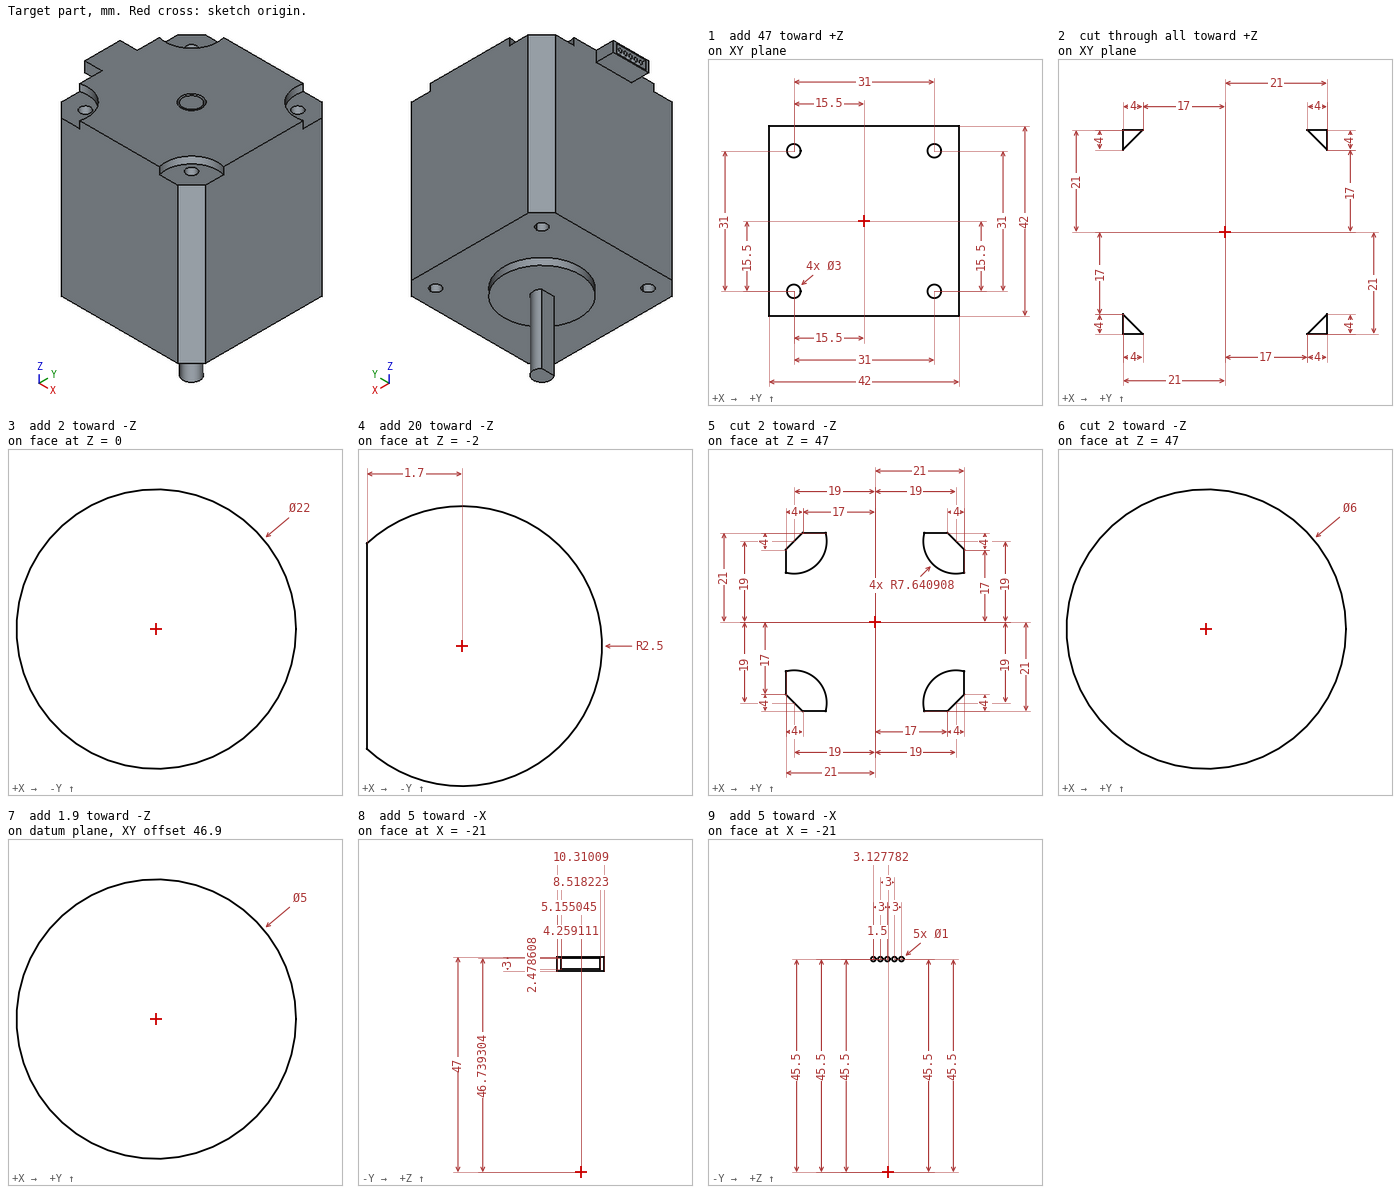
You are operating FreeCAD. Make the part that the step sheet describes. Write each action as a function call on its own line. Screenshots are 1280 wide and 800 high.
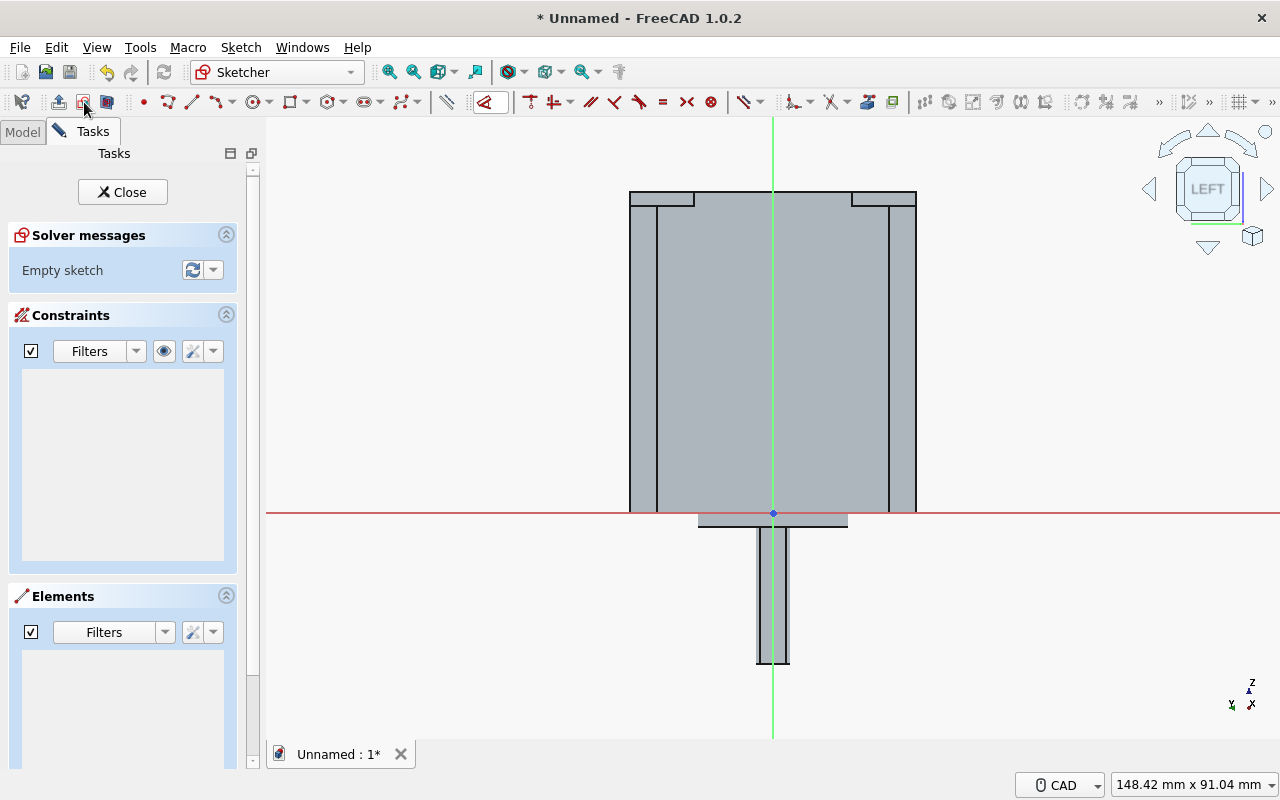
scroll(782, 174, up, 11)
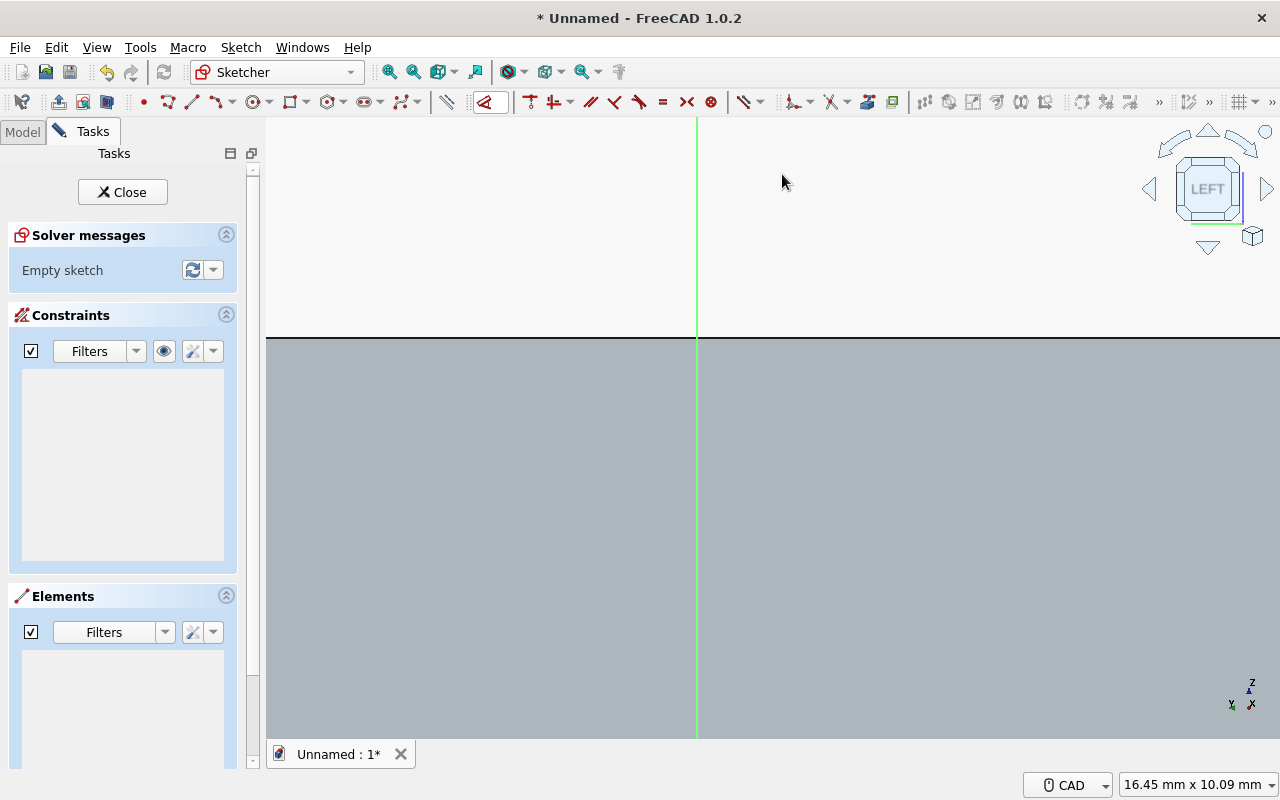
key(g)
key(r)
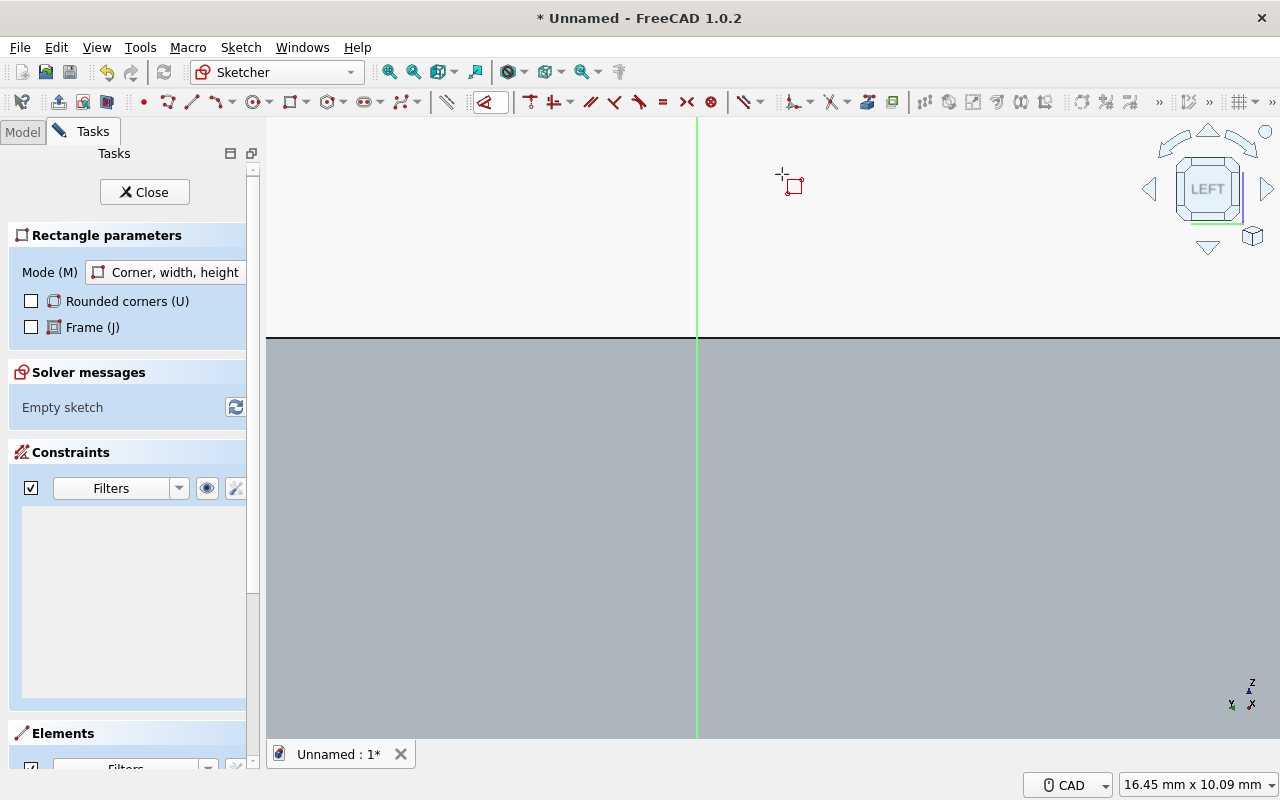
click(379, 338)
click(1015, 523)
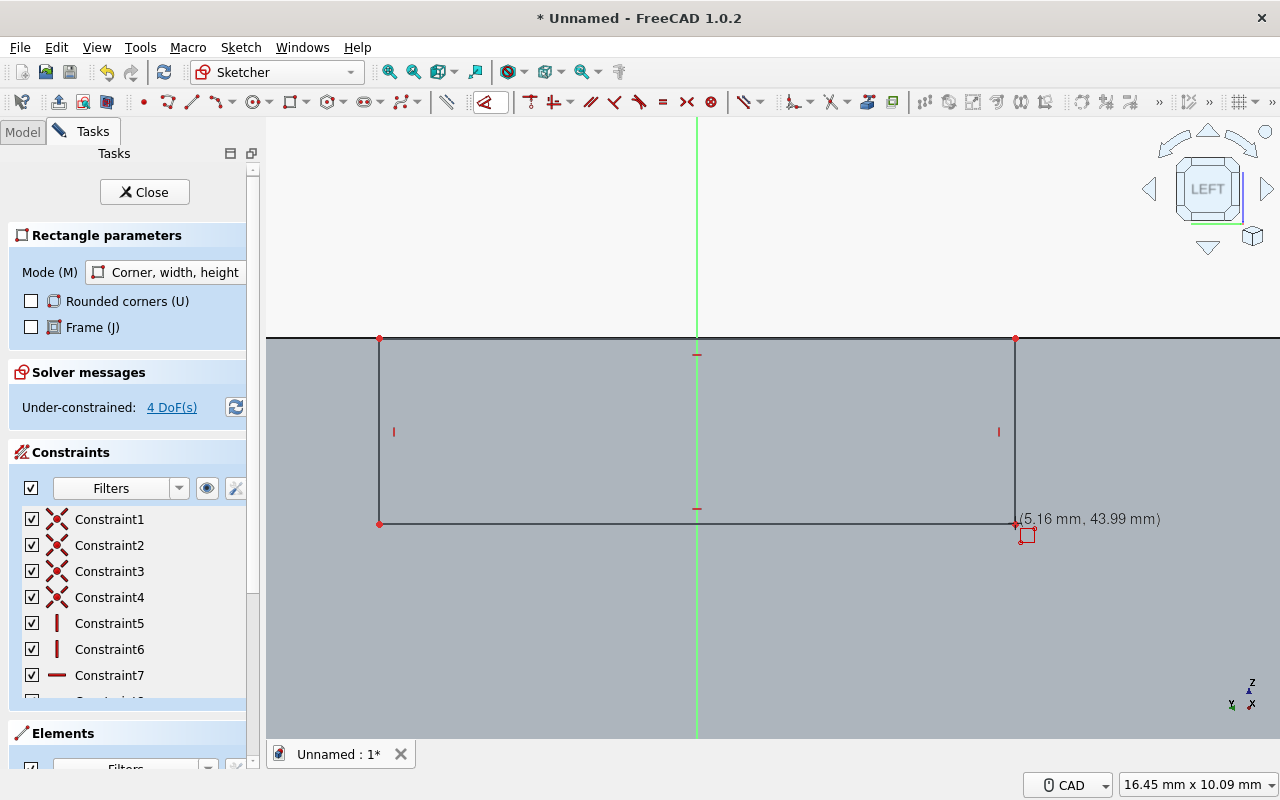
click(434, 355)
click(959, 507)
key(Escape)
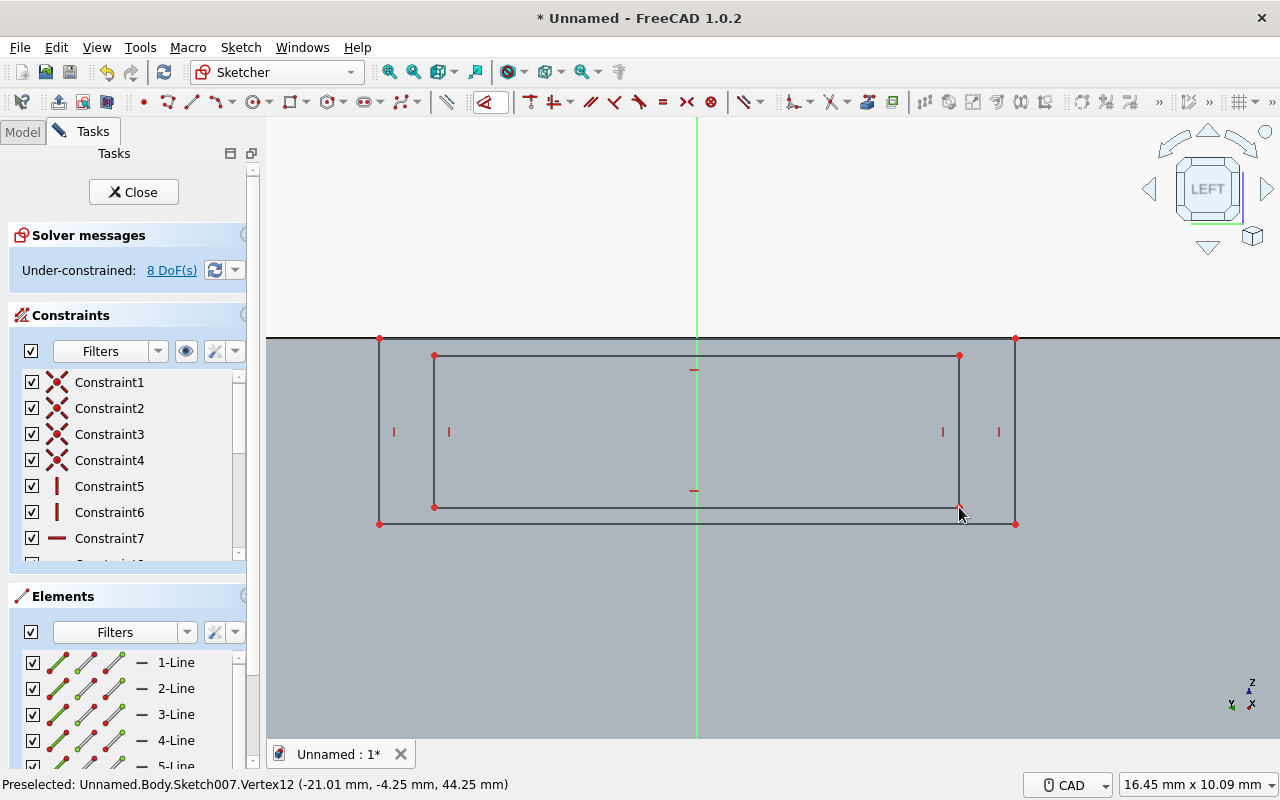
click(379, 394)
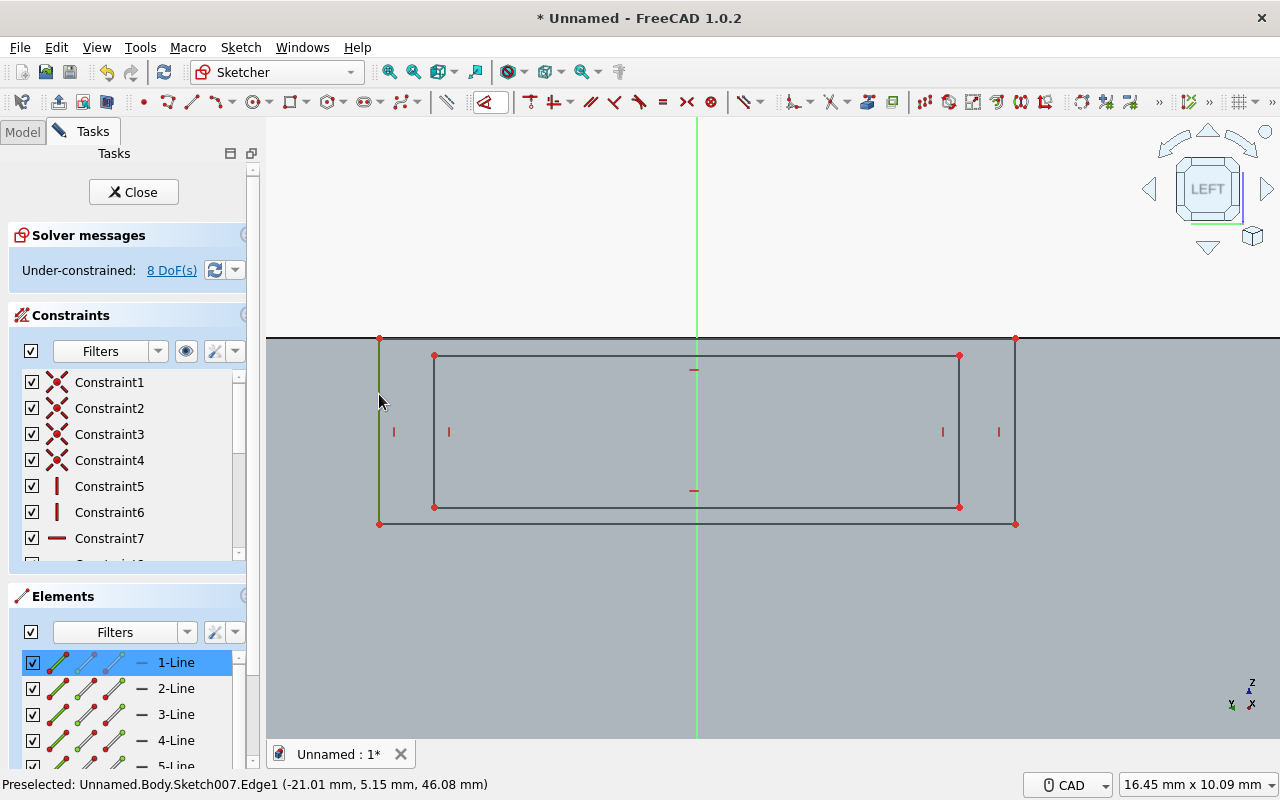
click(502, 102)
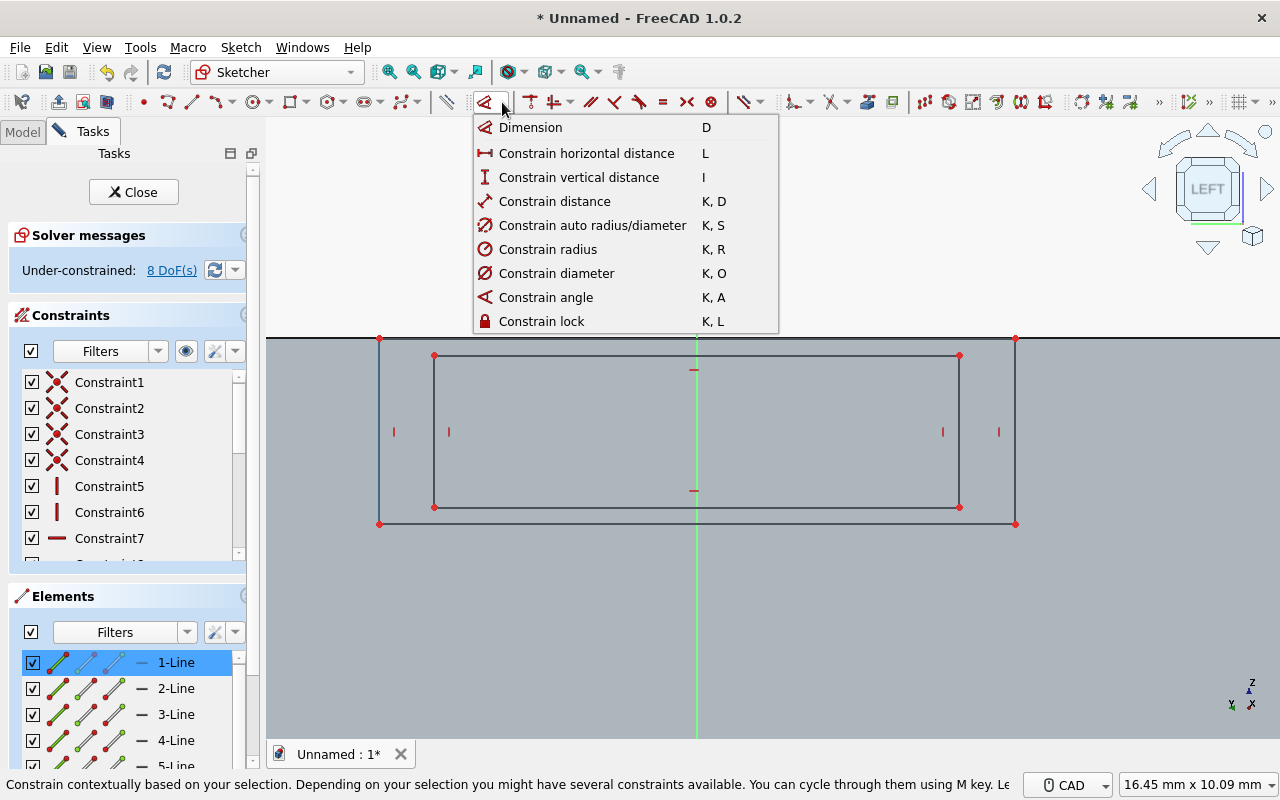
click(626, 177)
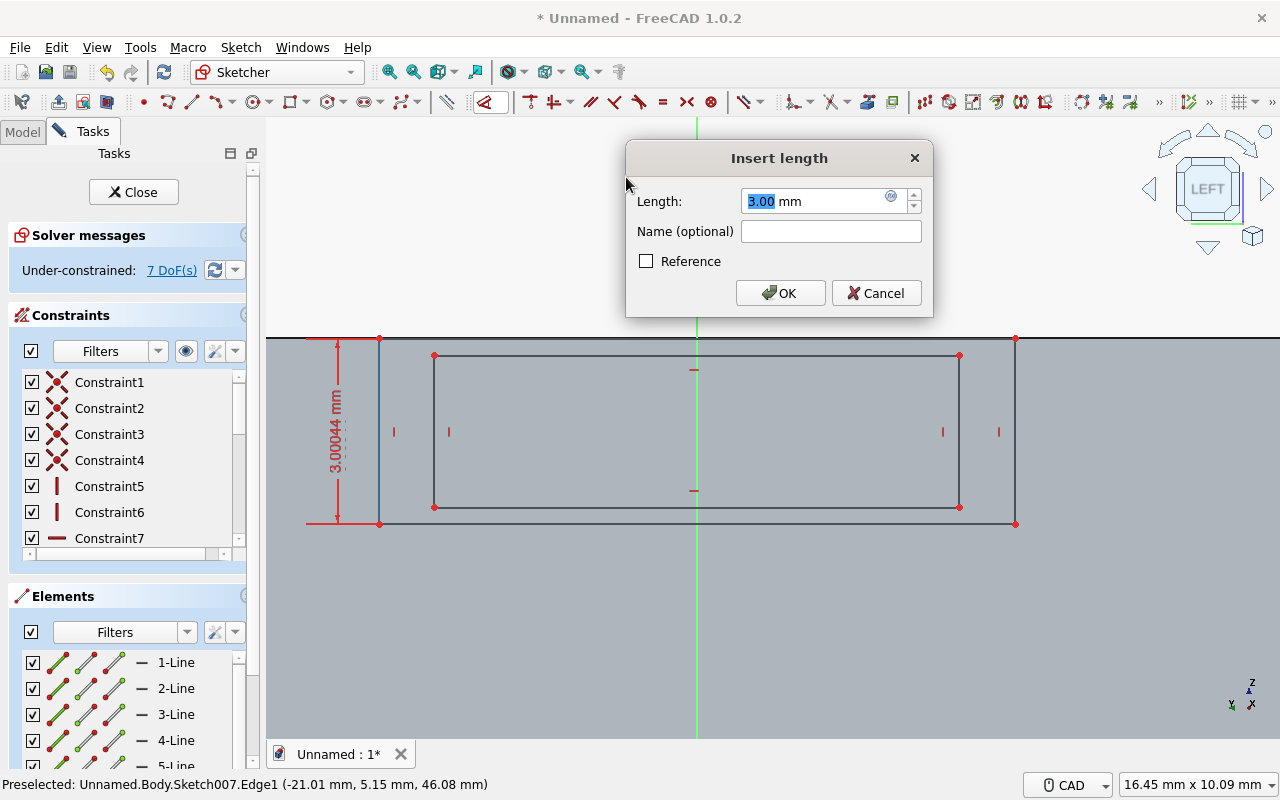
text(3)
key(Return)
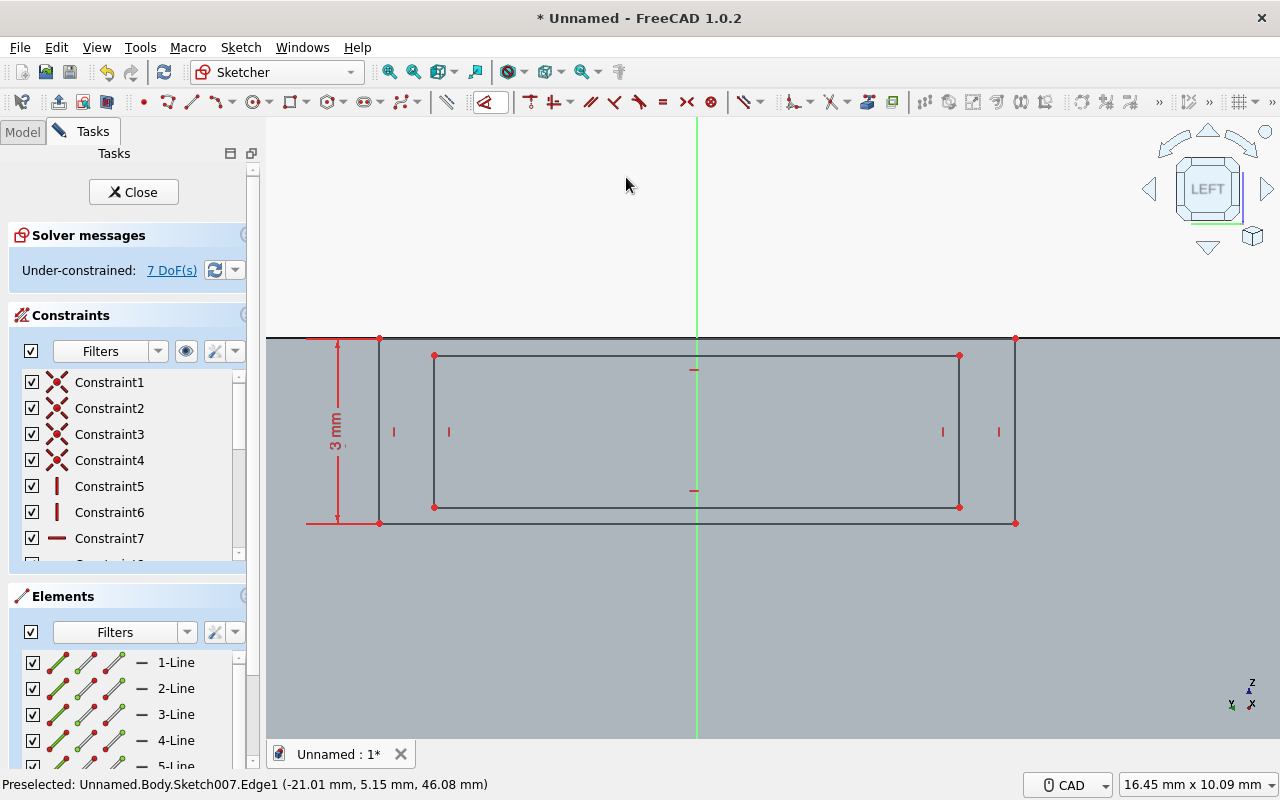
click(379, 339)